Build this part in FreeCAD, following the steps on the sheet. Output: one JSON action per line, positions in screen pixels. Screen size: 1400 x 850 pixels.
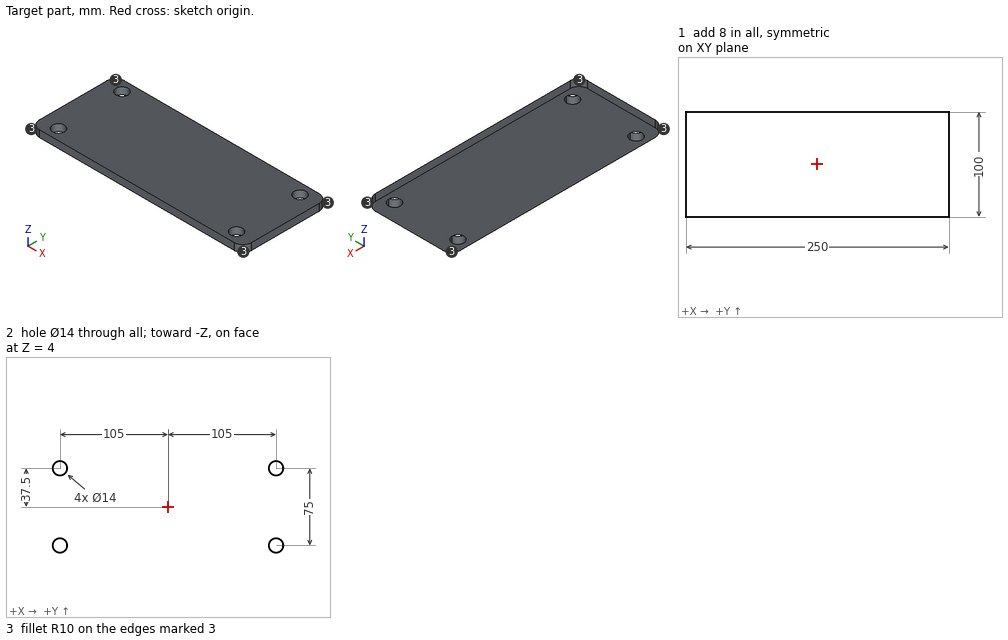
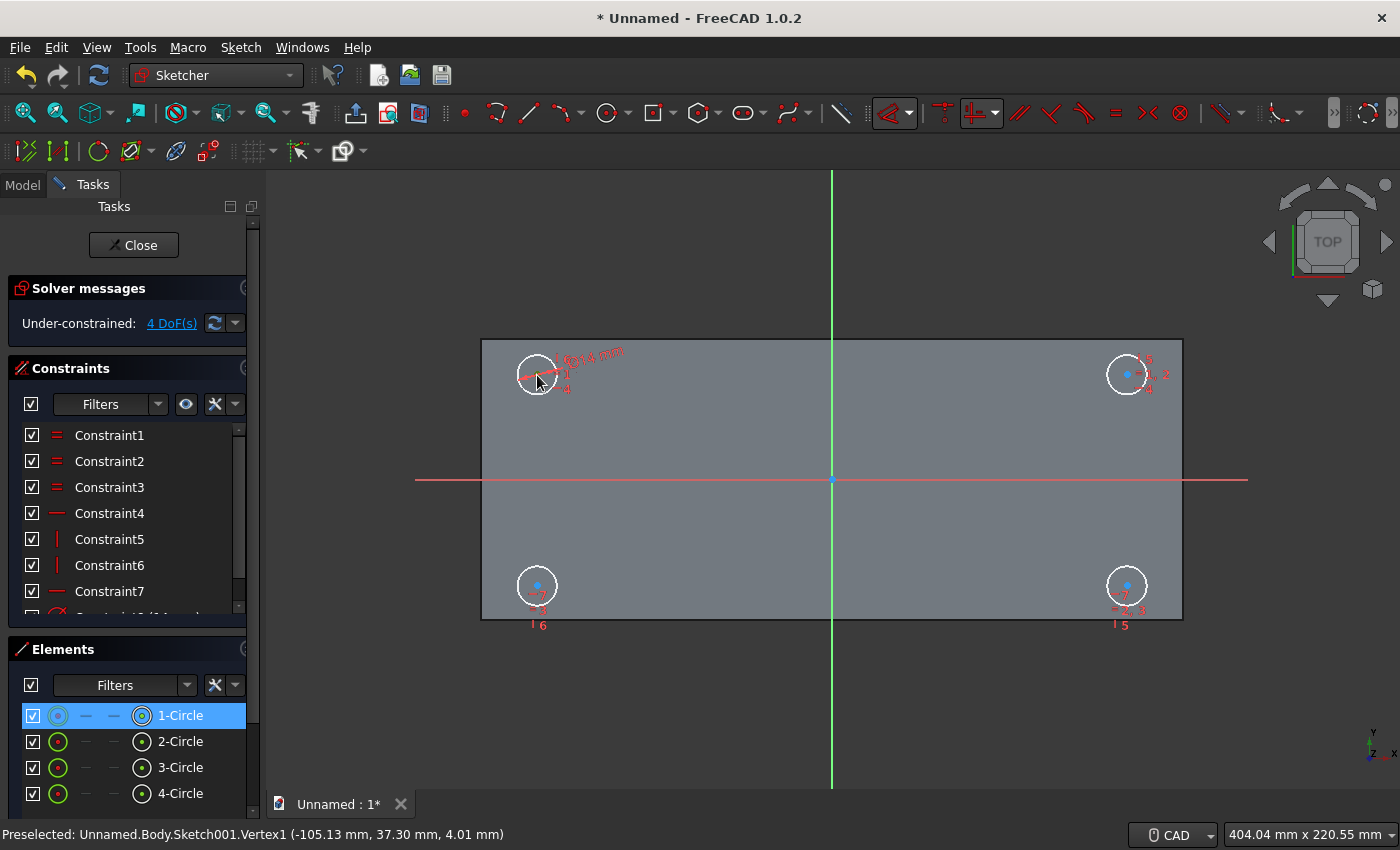
{"action": "left_click", "coordinate": [912, 114]}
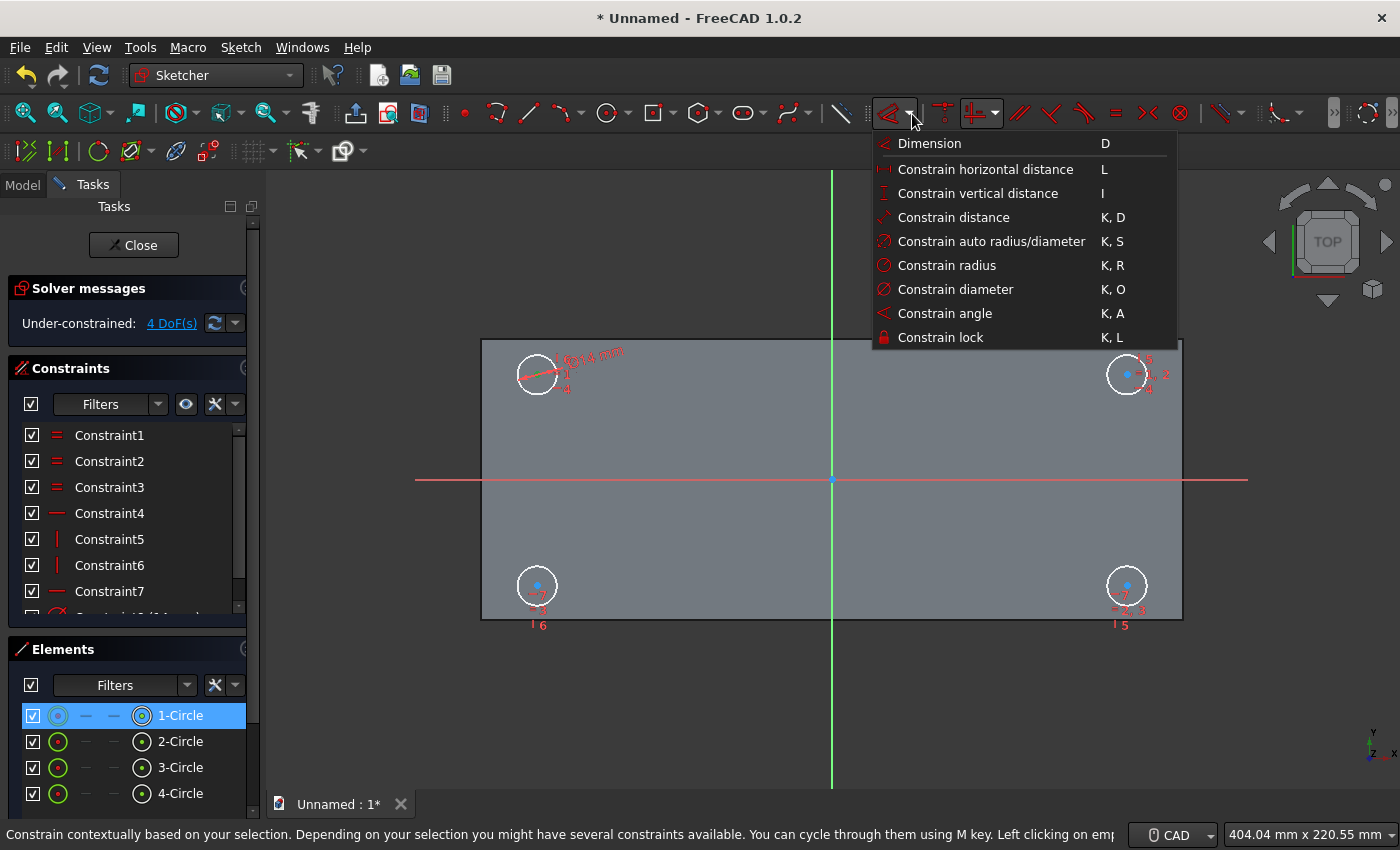
{"action": "left_click", "coordinate": [1025, 169]}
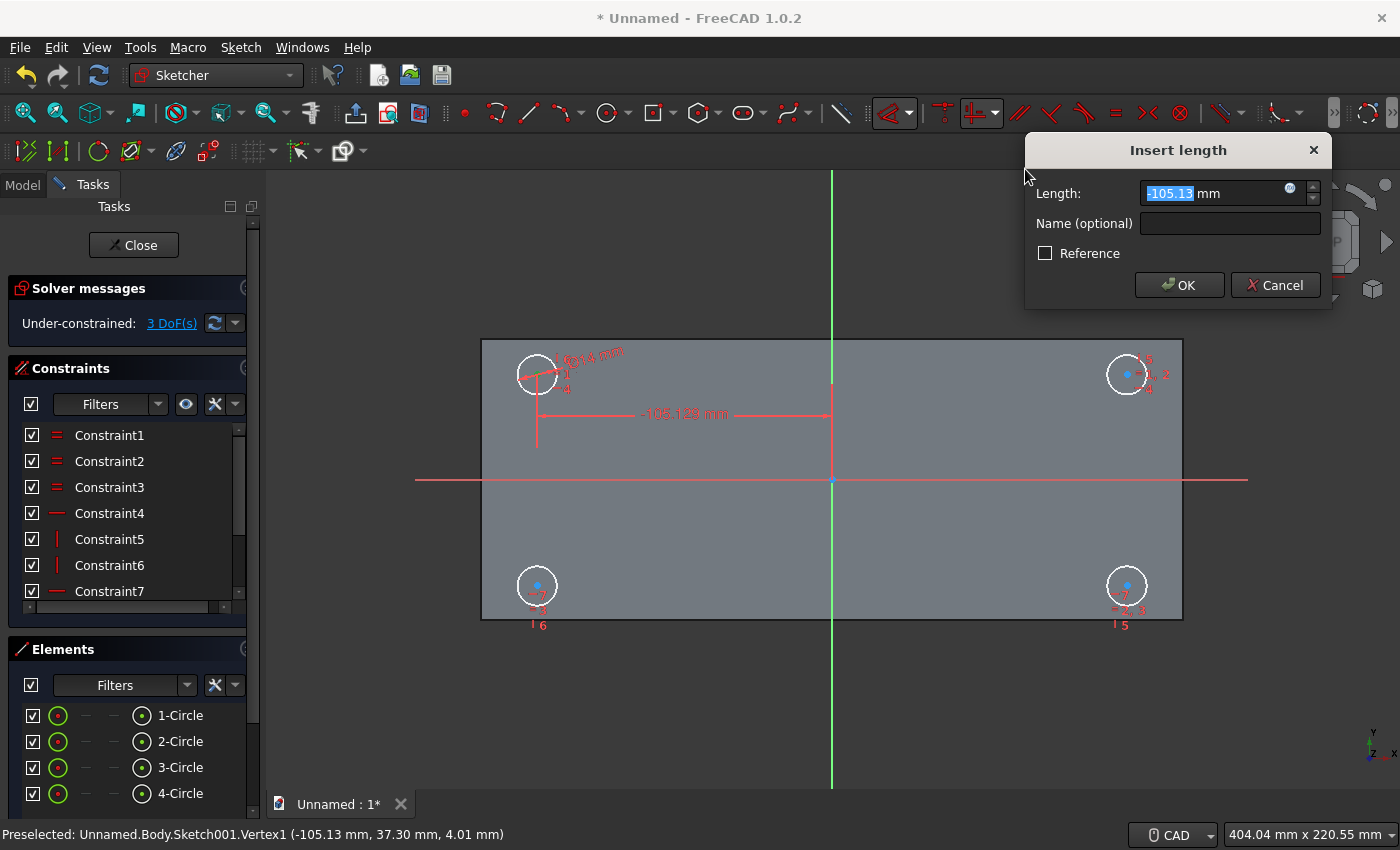
{"action": "type", "text": "-105"}
{"action": "key", "text": "Return"}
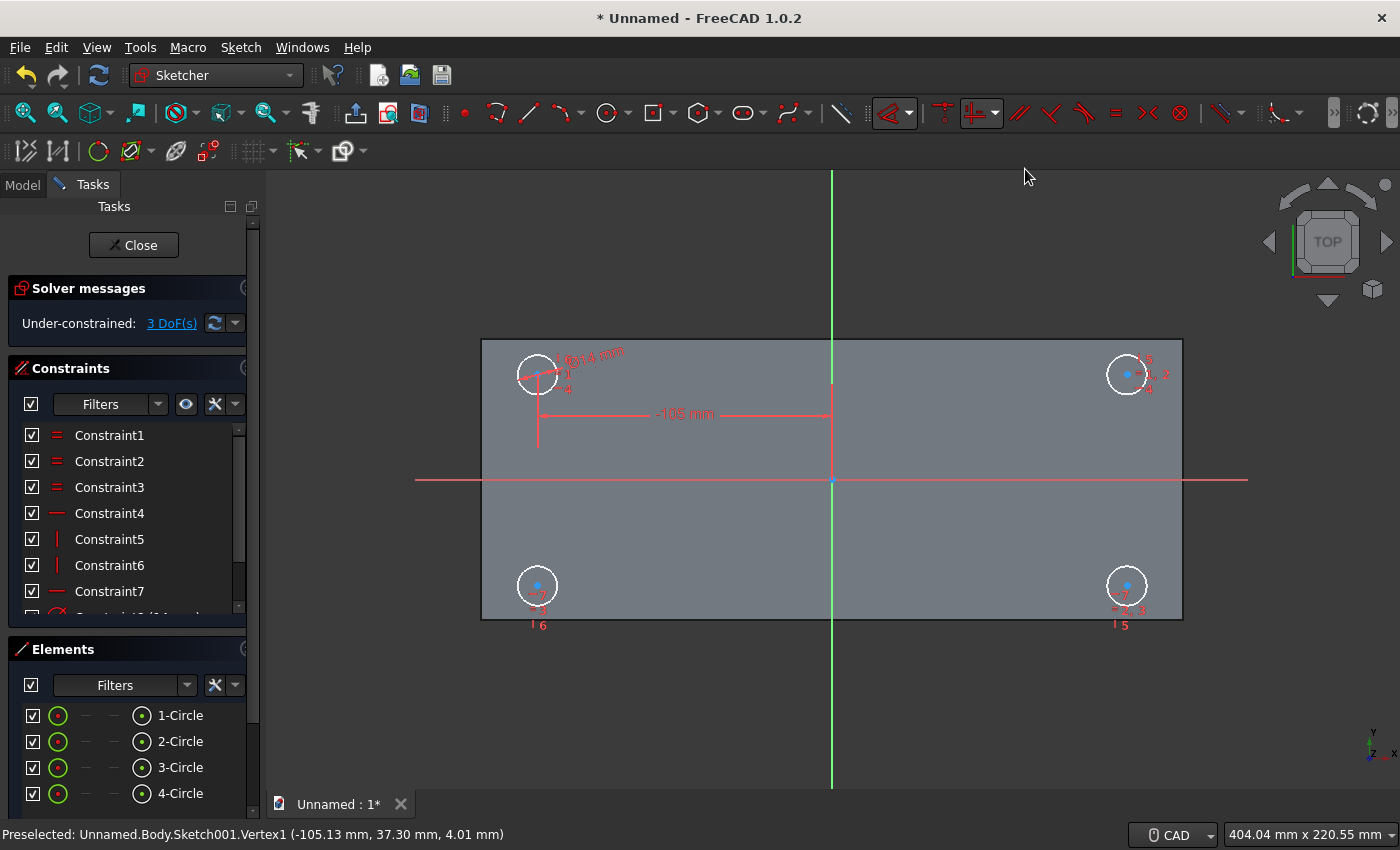
{"action": "left_click", "coordinate": [1127, 375]}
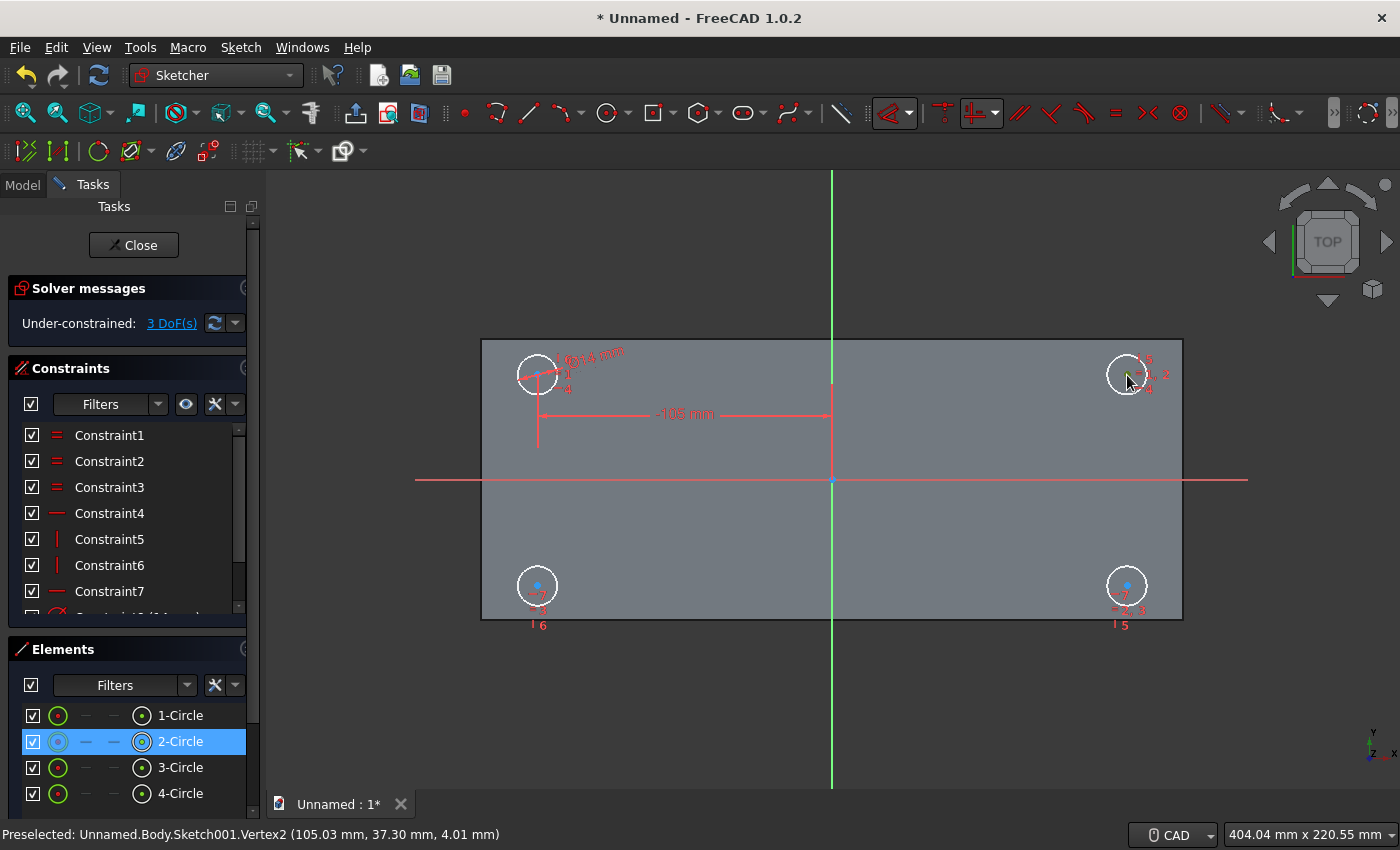
{"action": "left_click", "coordinate": [912, 114]}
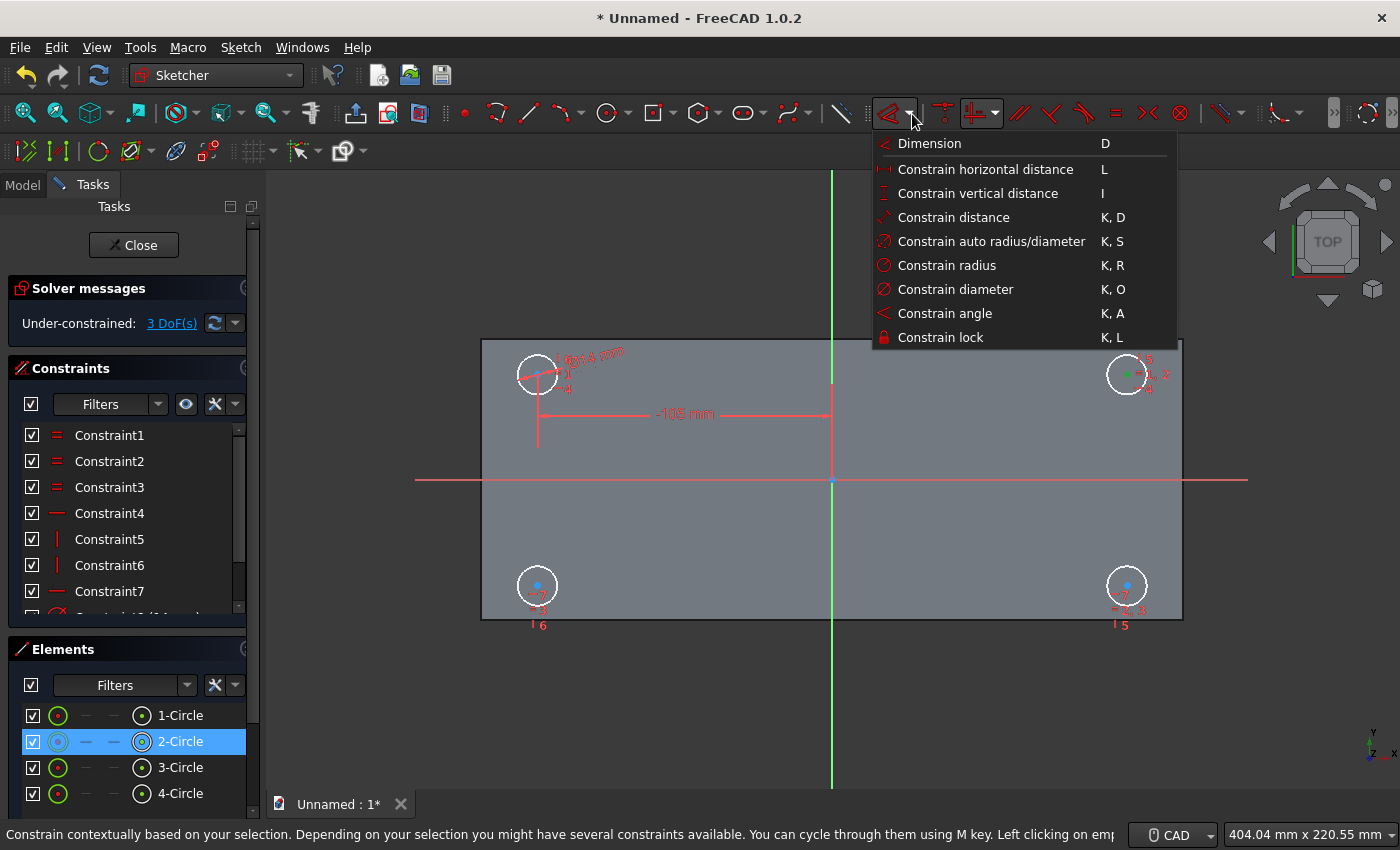
{"action": "left_click", "coordinate": [1025, 169]}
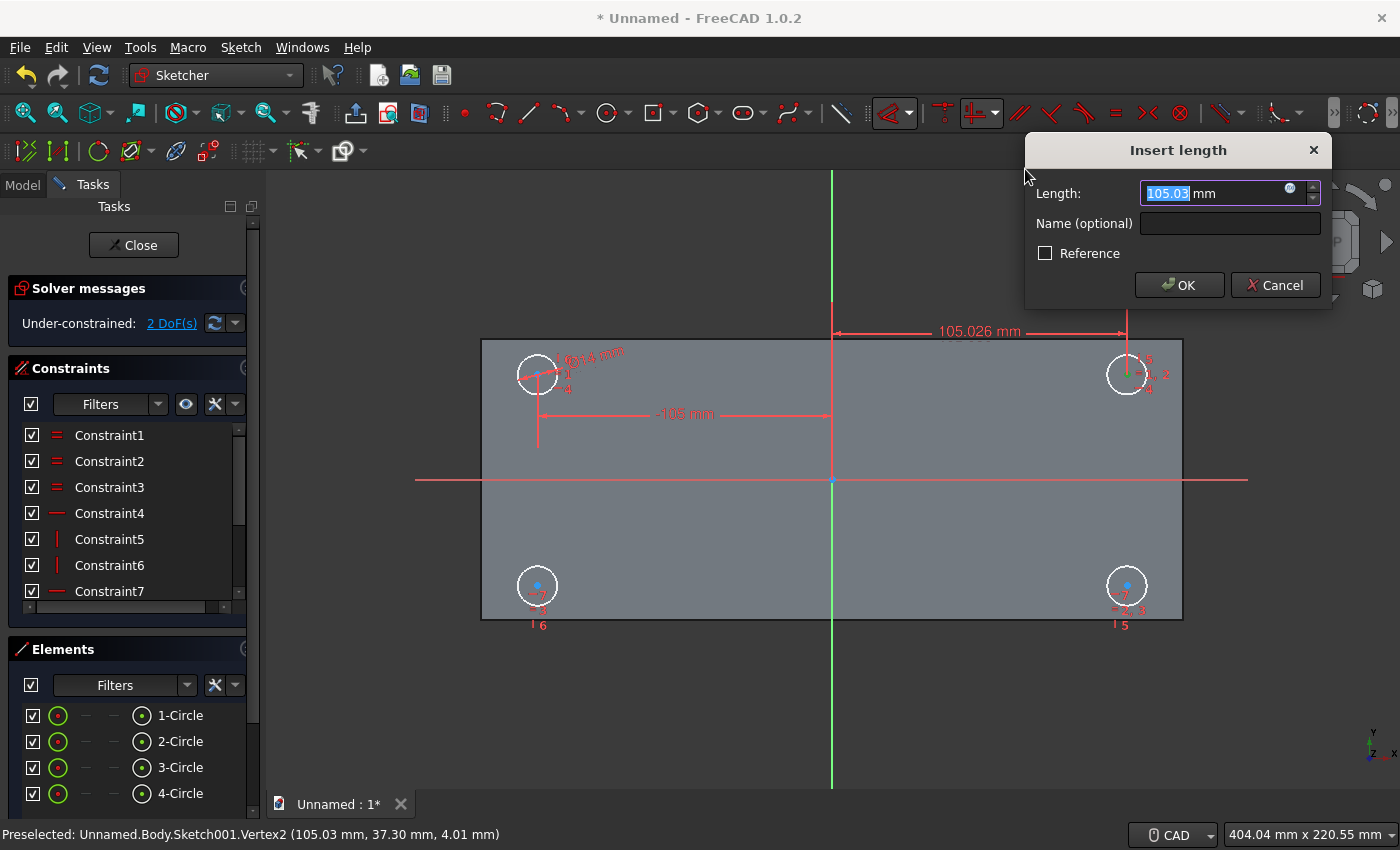
{"action": "type", "text": "105"}
{"action": "key", "text": "Return"}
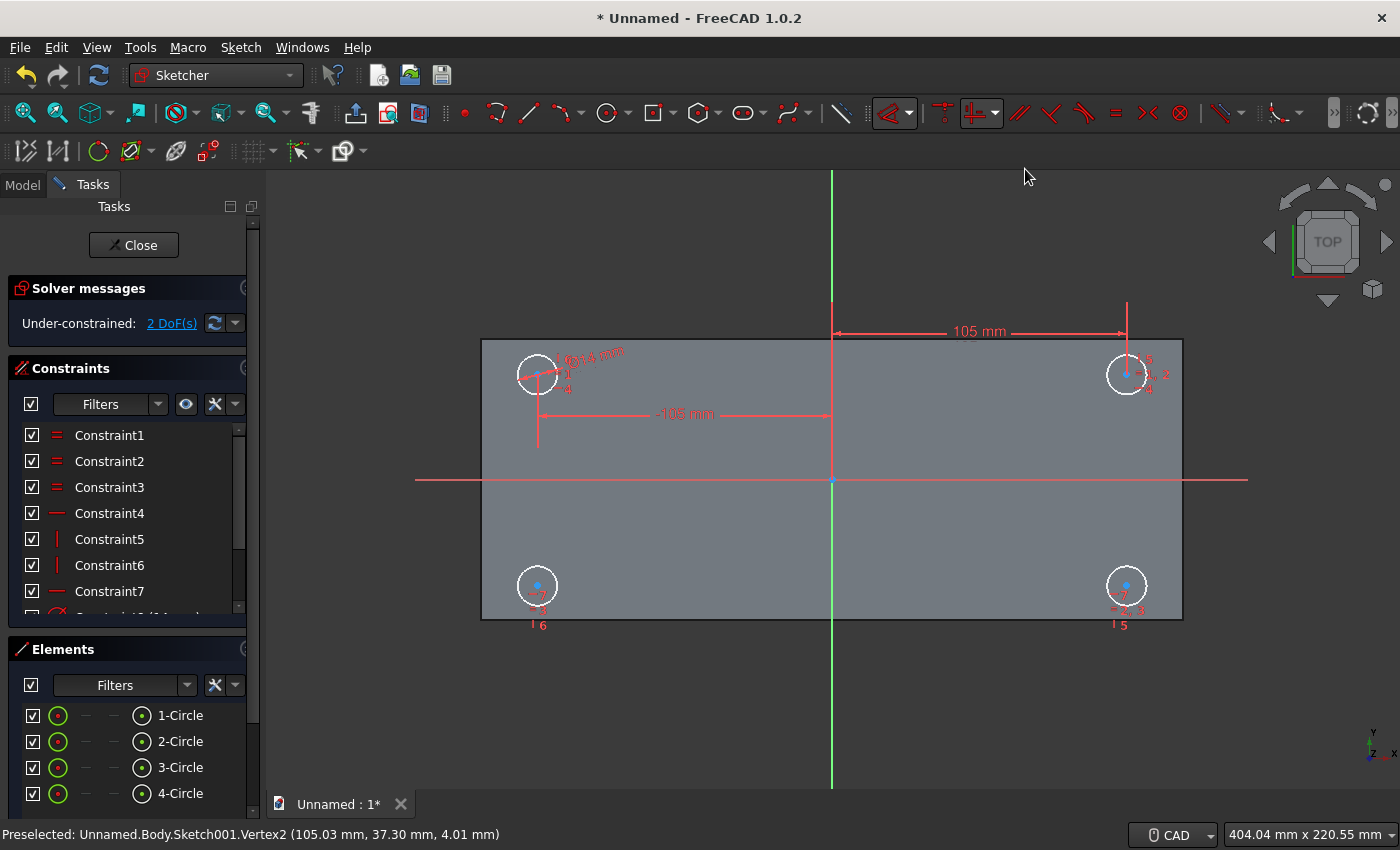
{"action": "left_click", "coordinate": [1127, 375]}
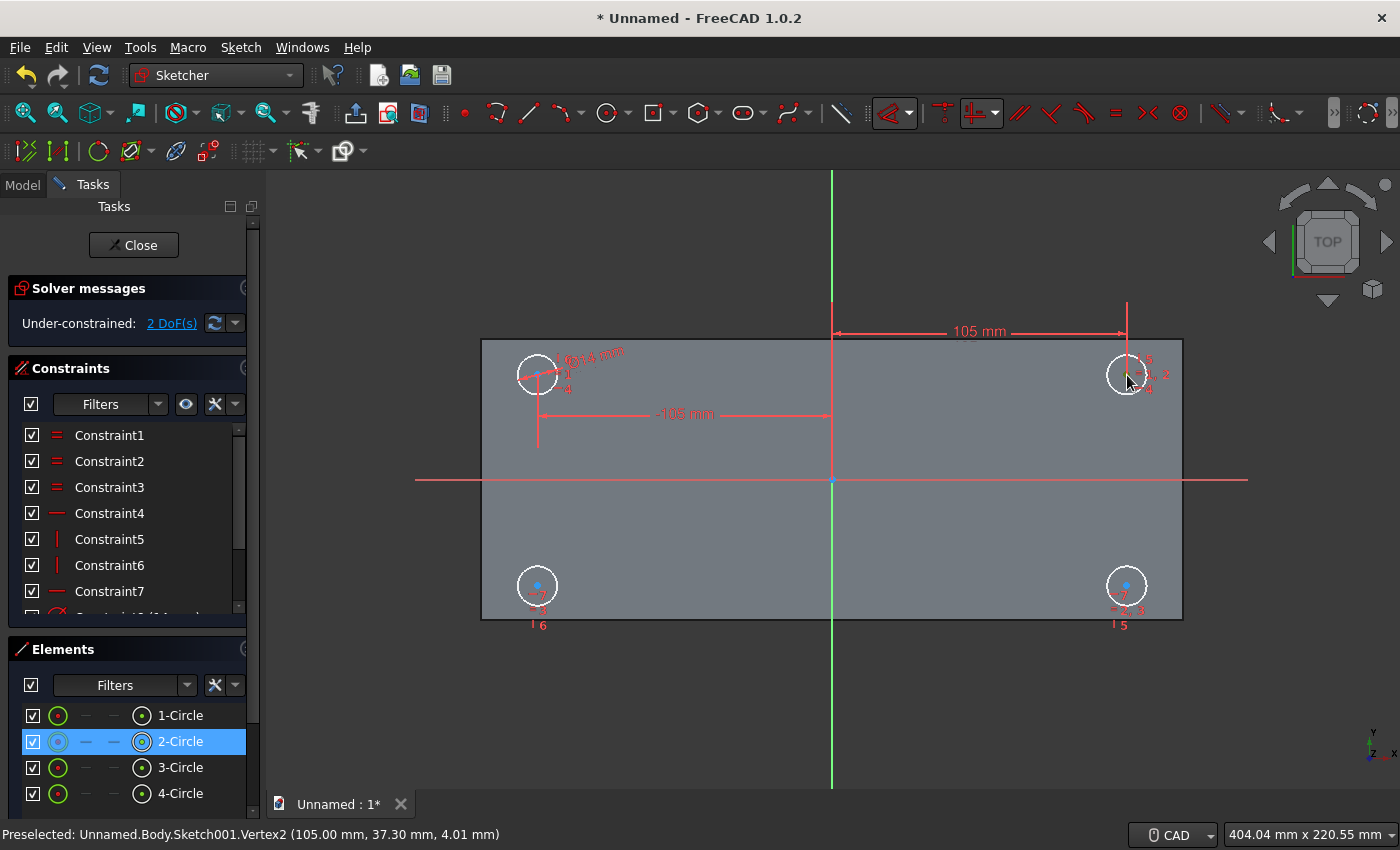
{"action": "left_click", "coordinate": [1127, 586]}